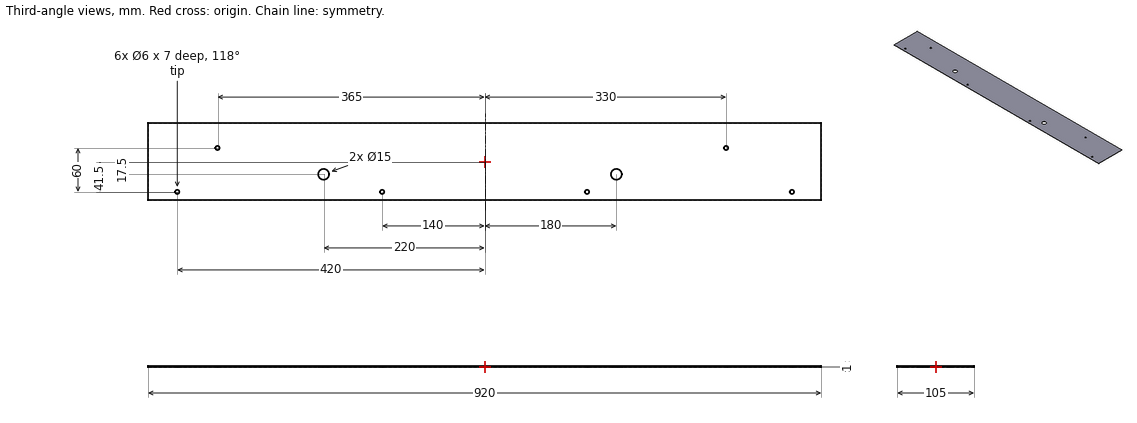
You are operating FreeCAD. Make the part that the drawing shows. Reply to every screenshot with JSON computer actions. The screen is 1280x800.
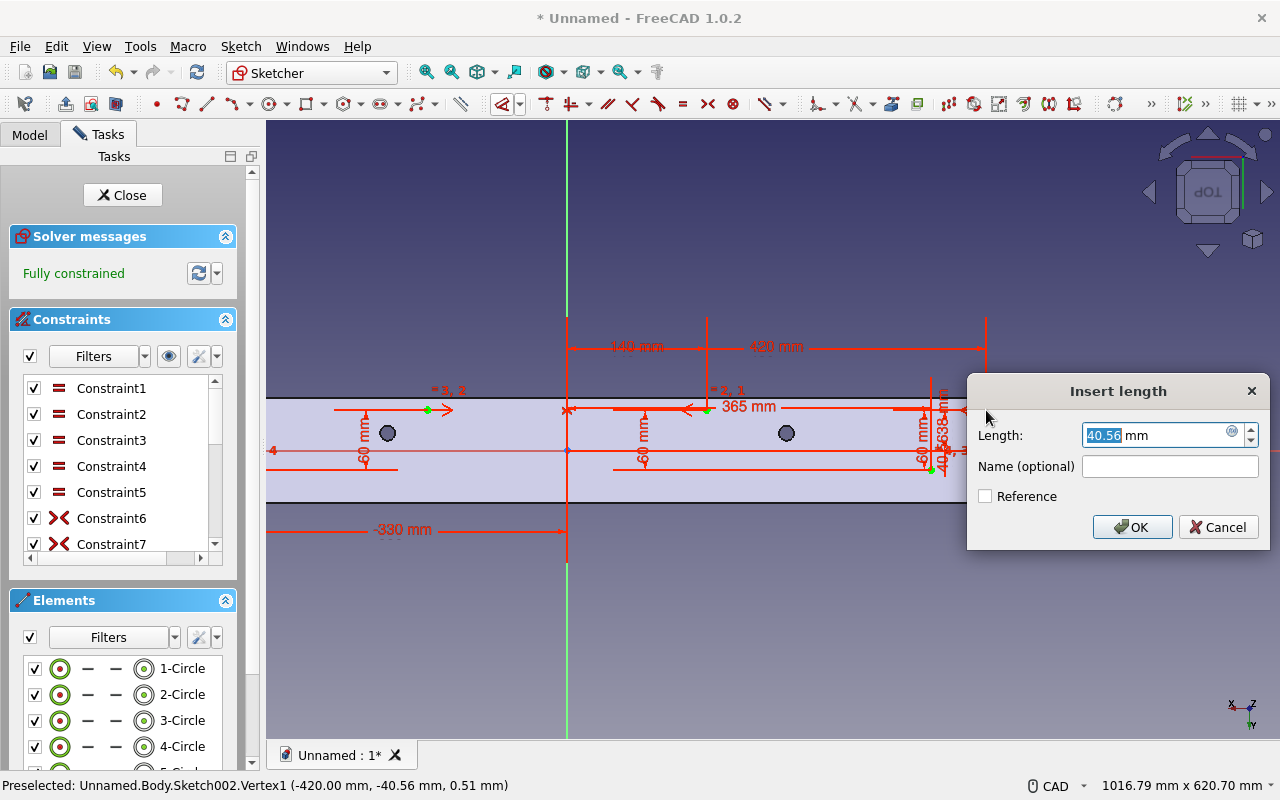
{"action": "type", "text": "41.5"}
{"action": "key", "text": "Return"}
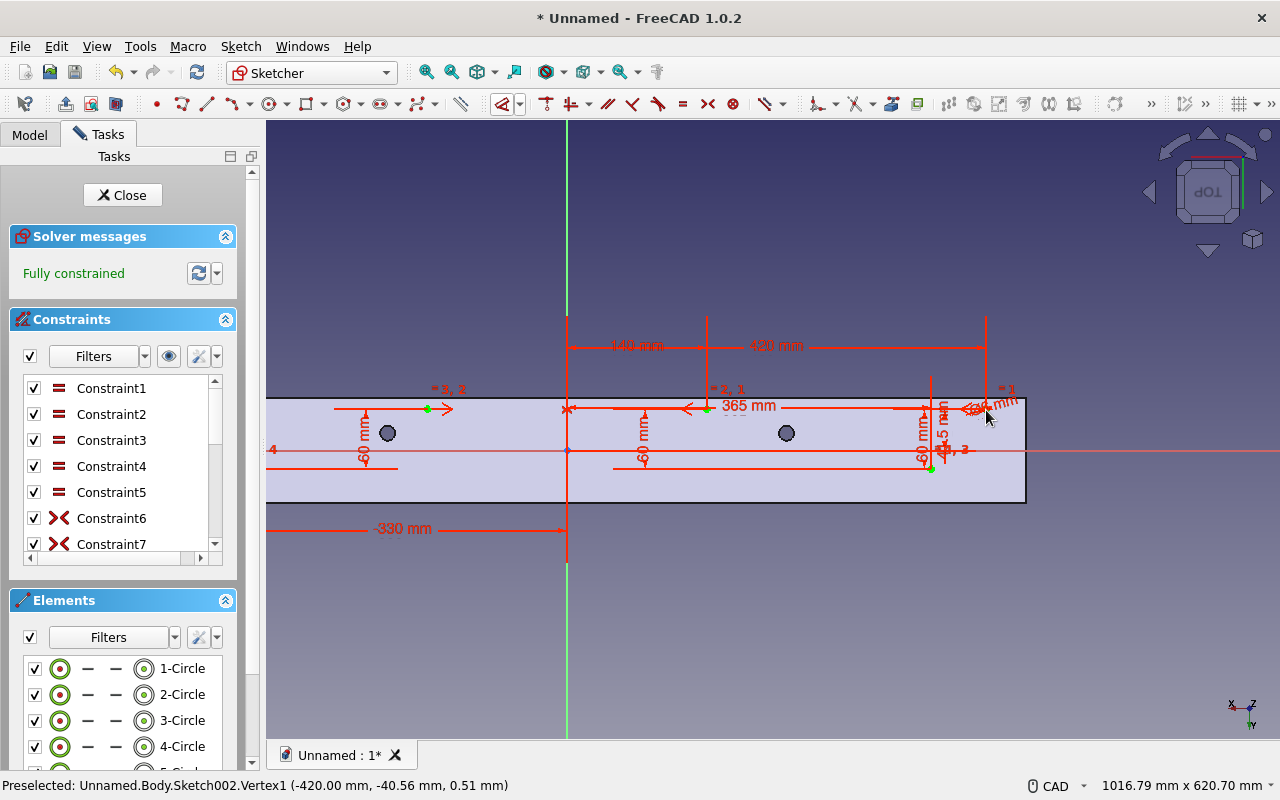
{"action": "left_click", "coordinate": [123, 195]}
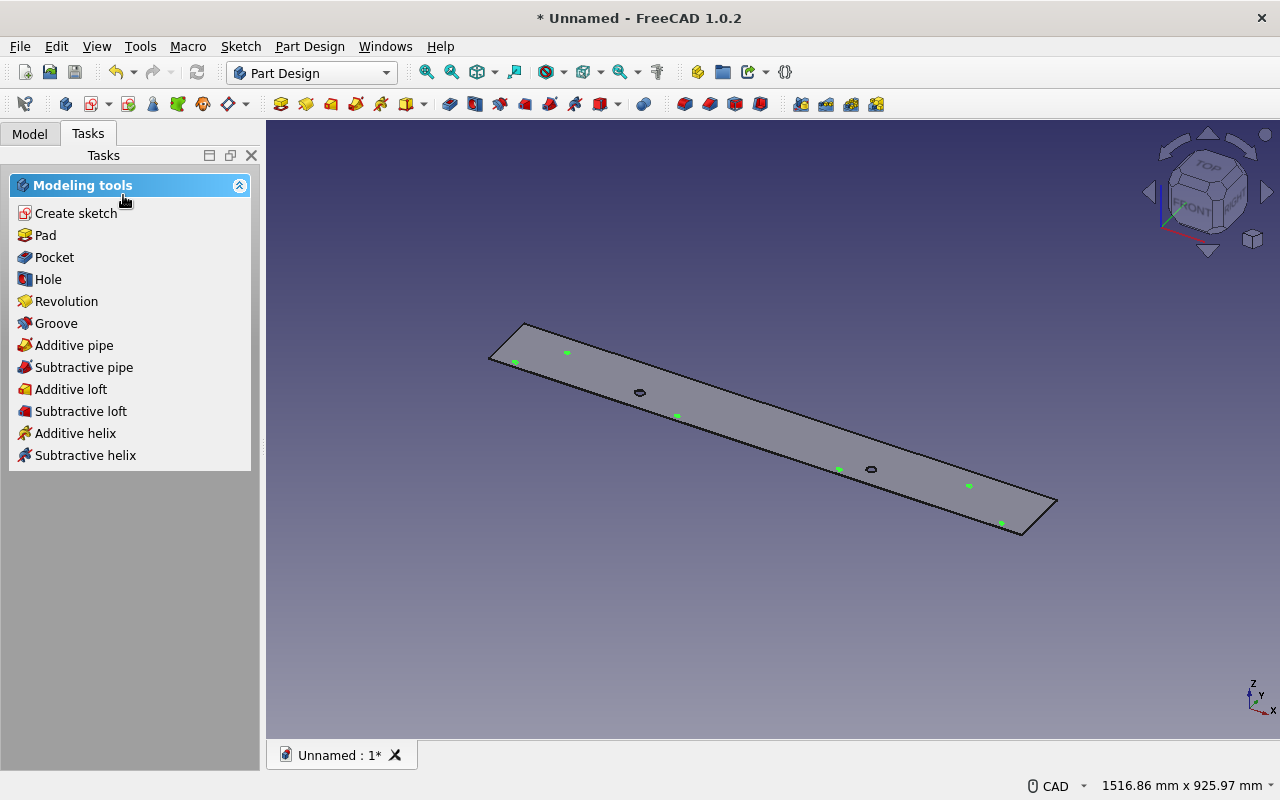
{"action": "left_click", "coordinate": [475, 104]}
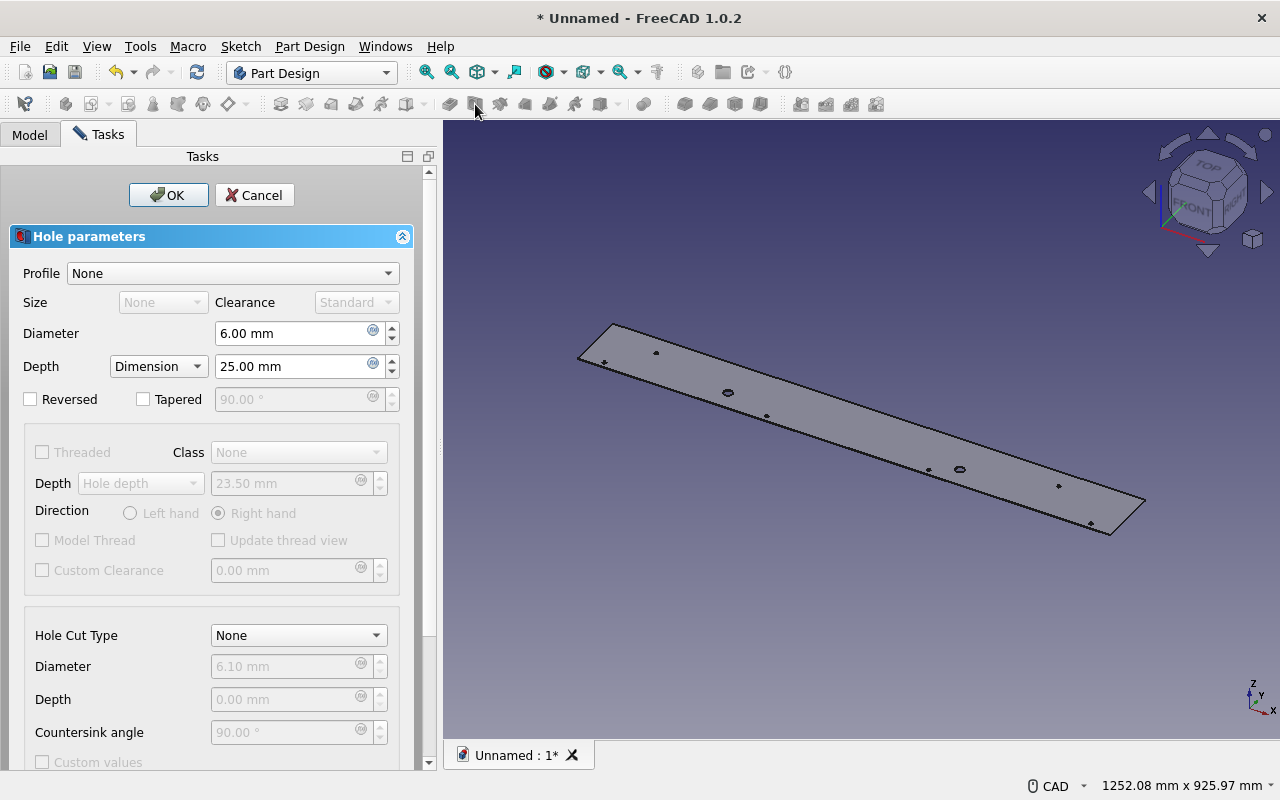
{"action": "triple_click", "coordinate": [300, 334]}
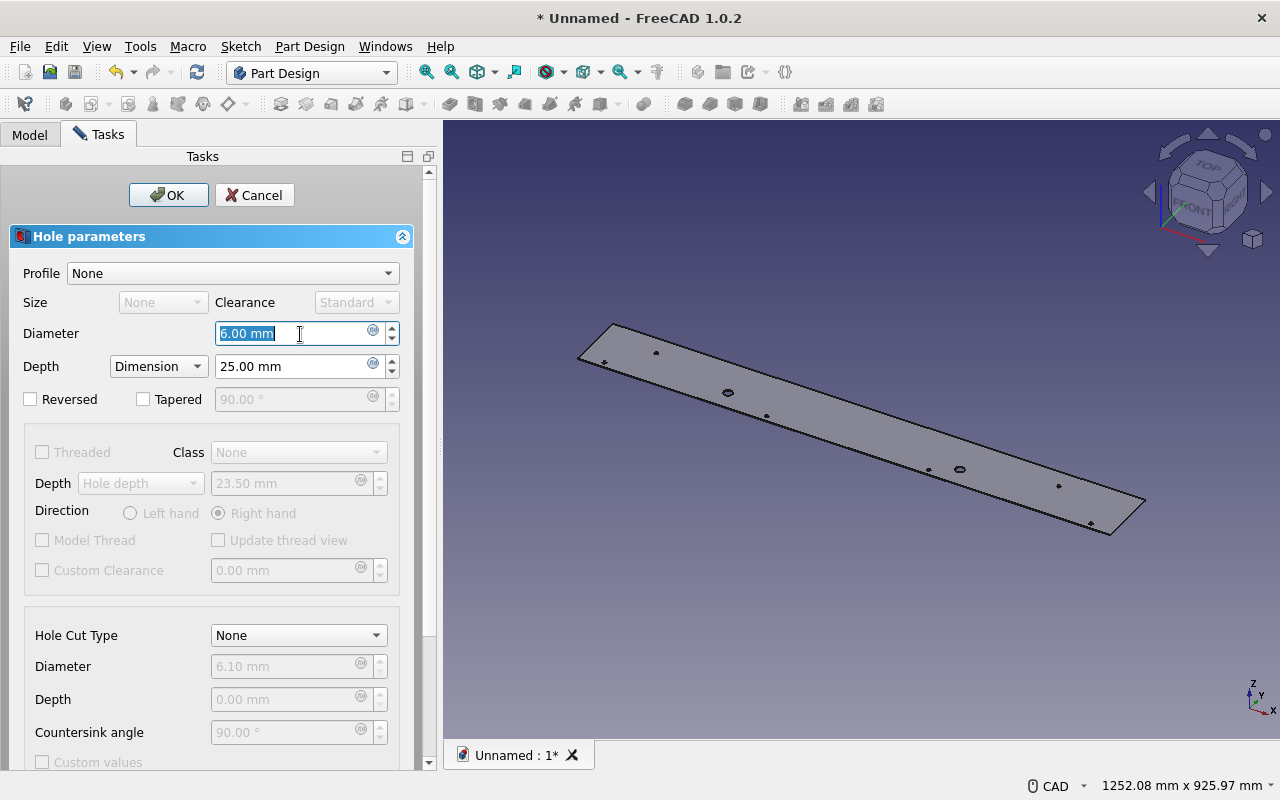
{"action": "type", "text": "6"}
{"action": "key", "text": "Tab"}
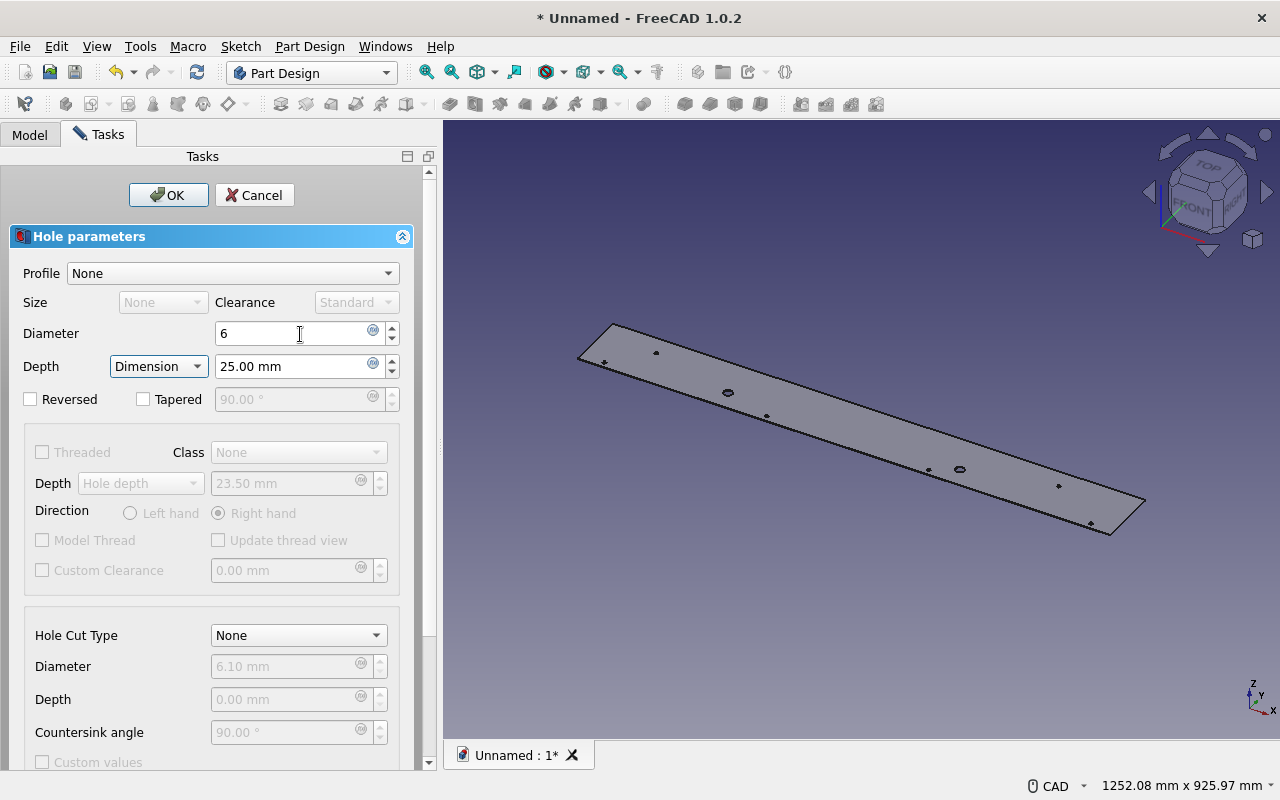
{"action": "triple_click", "coordinate": [300, 366]}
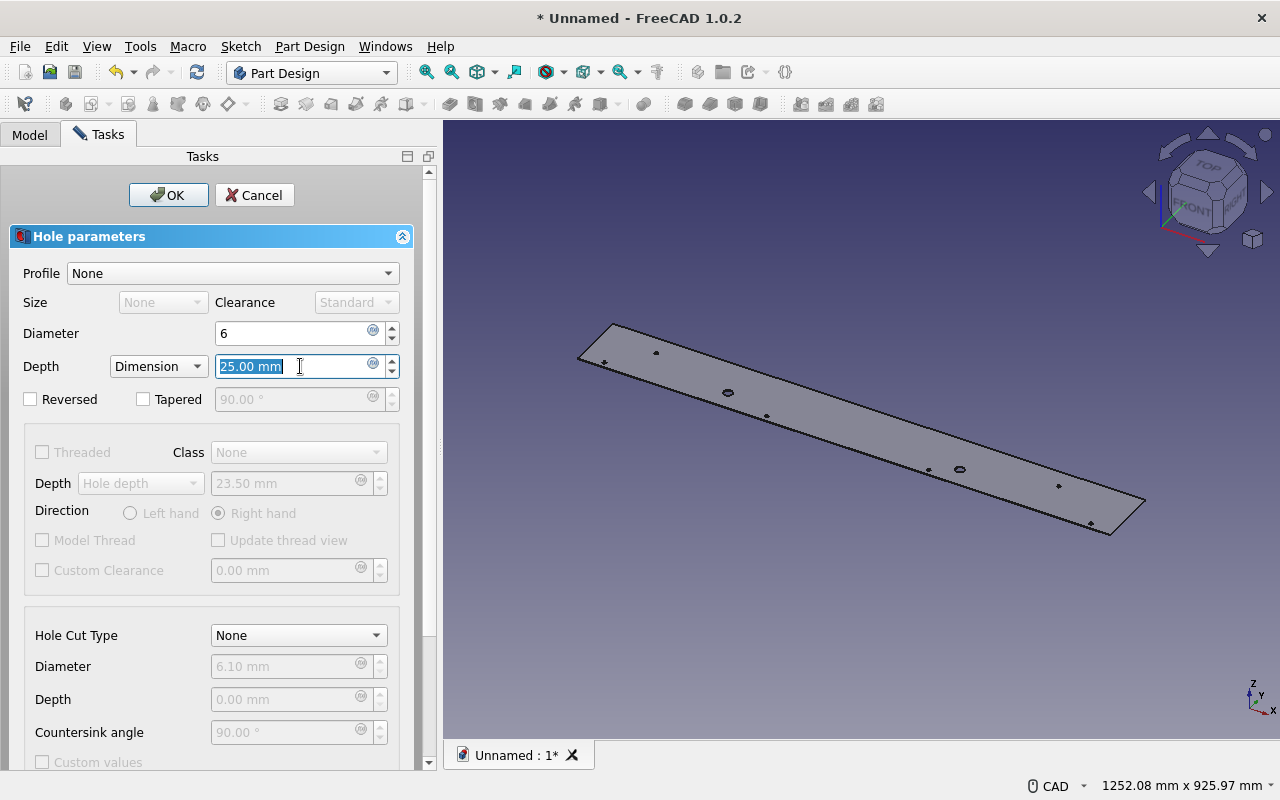
{"action": "type", "text": "7"}
{"action": "key", "text": "Tab"}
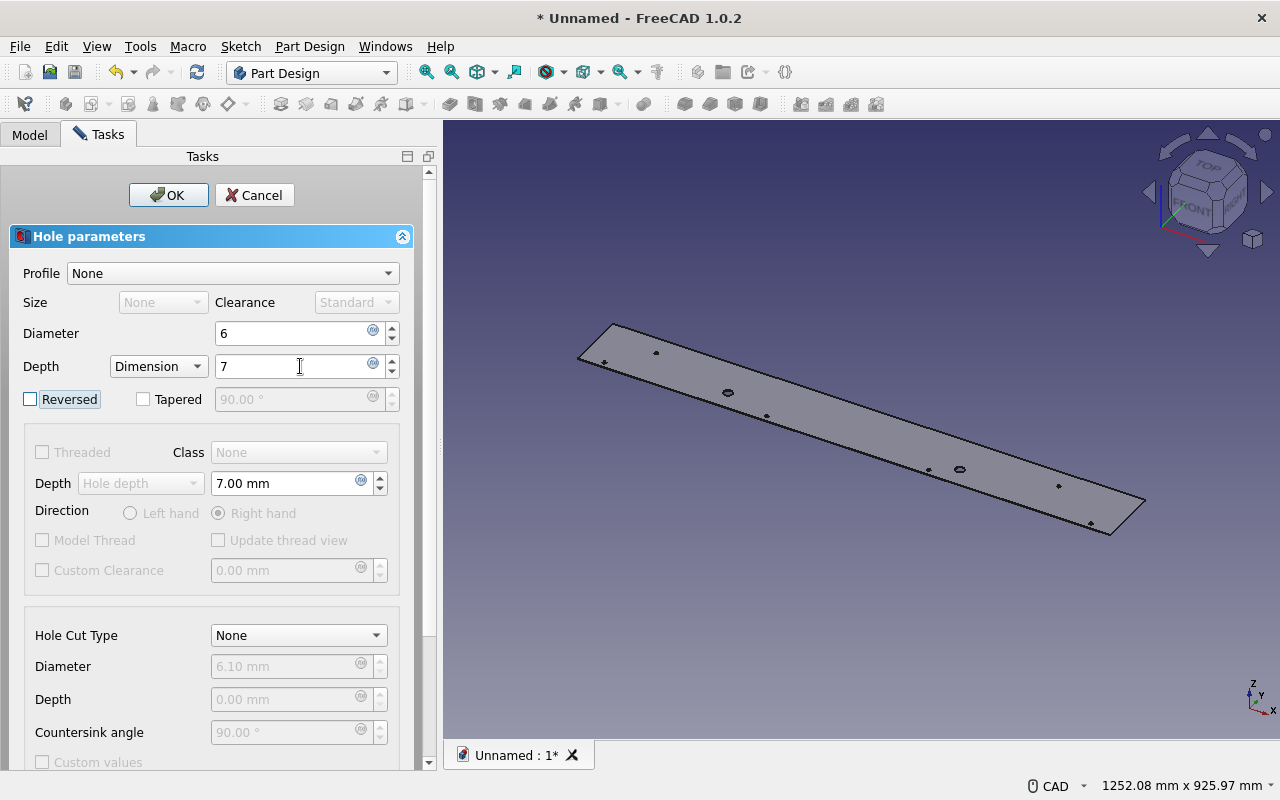
{"action": "left_click", "coordinate": [169, 195]}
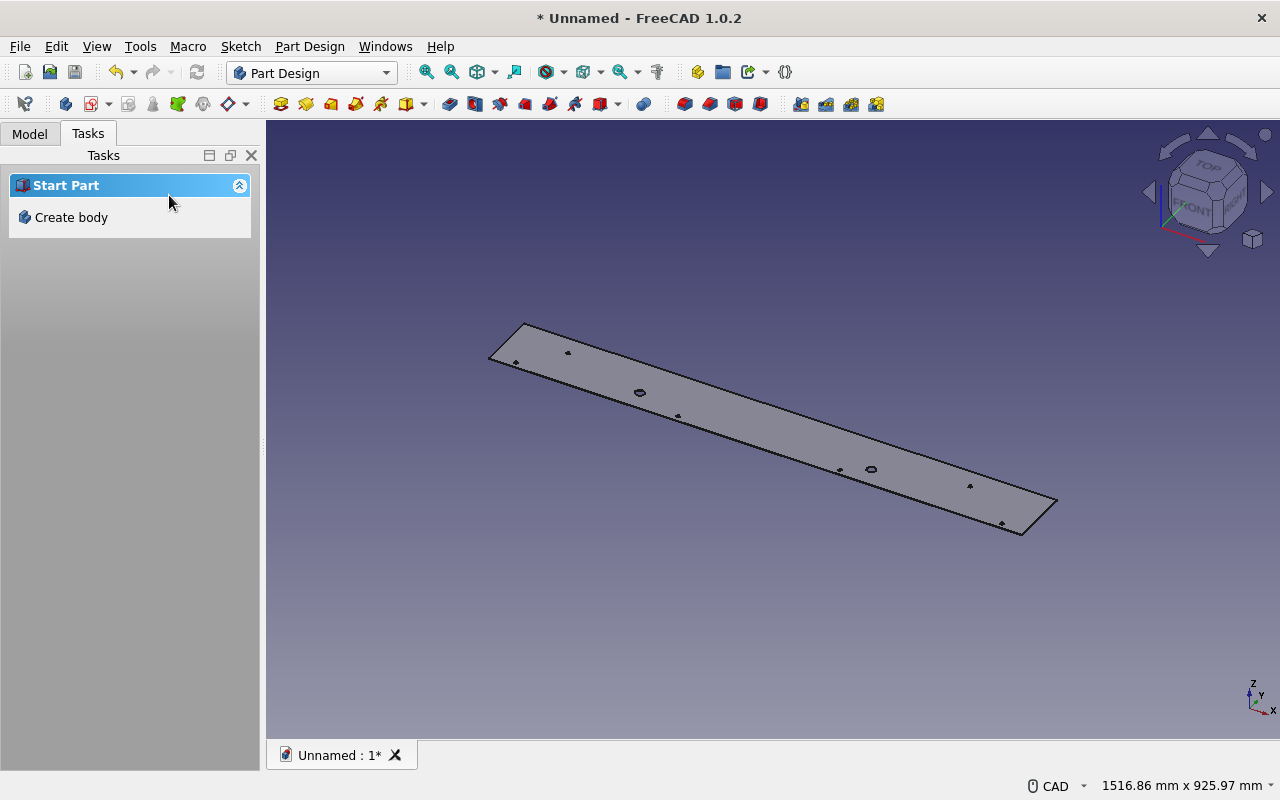
{"action": "key", "text": "0"}